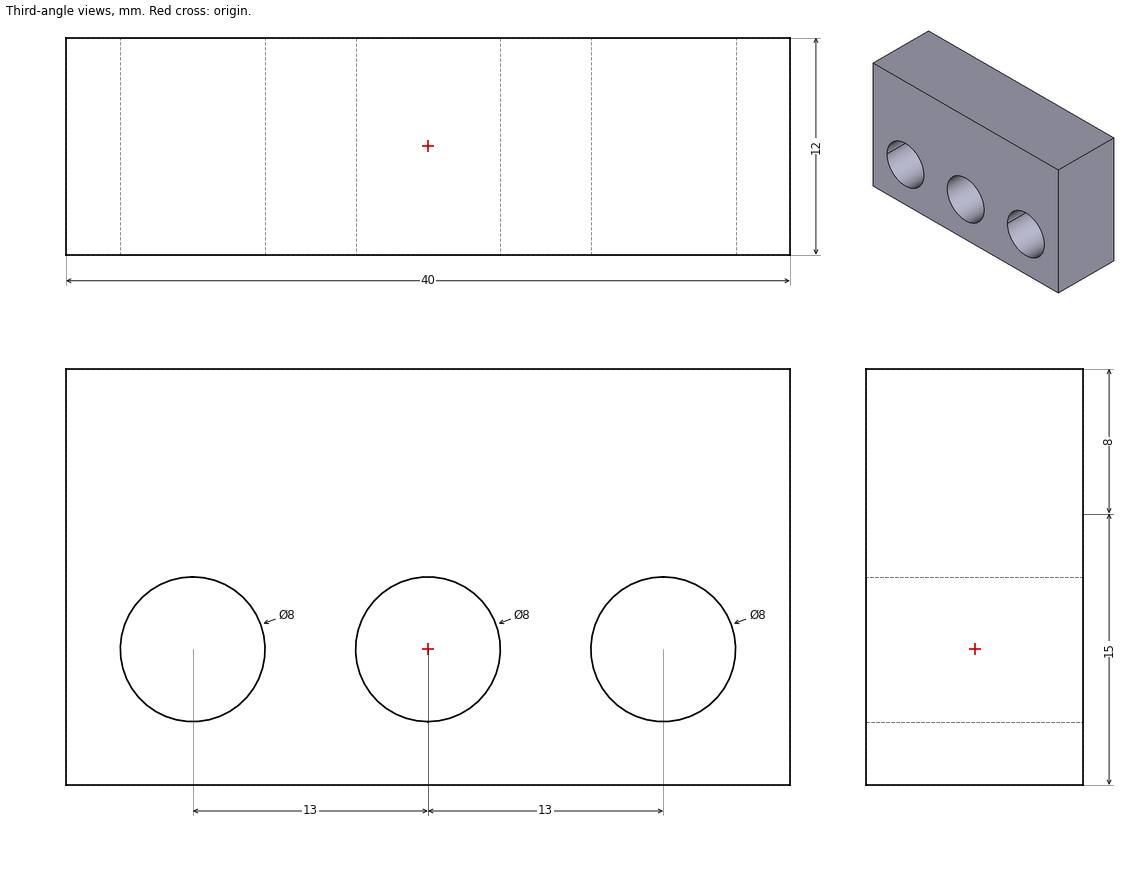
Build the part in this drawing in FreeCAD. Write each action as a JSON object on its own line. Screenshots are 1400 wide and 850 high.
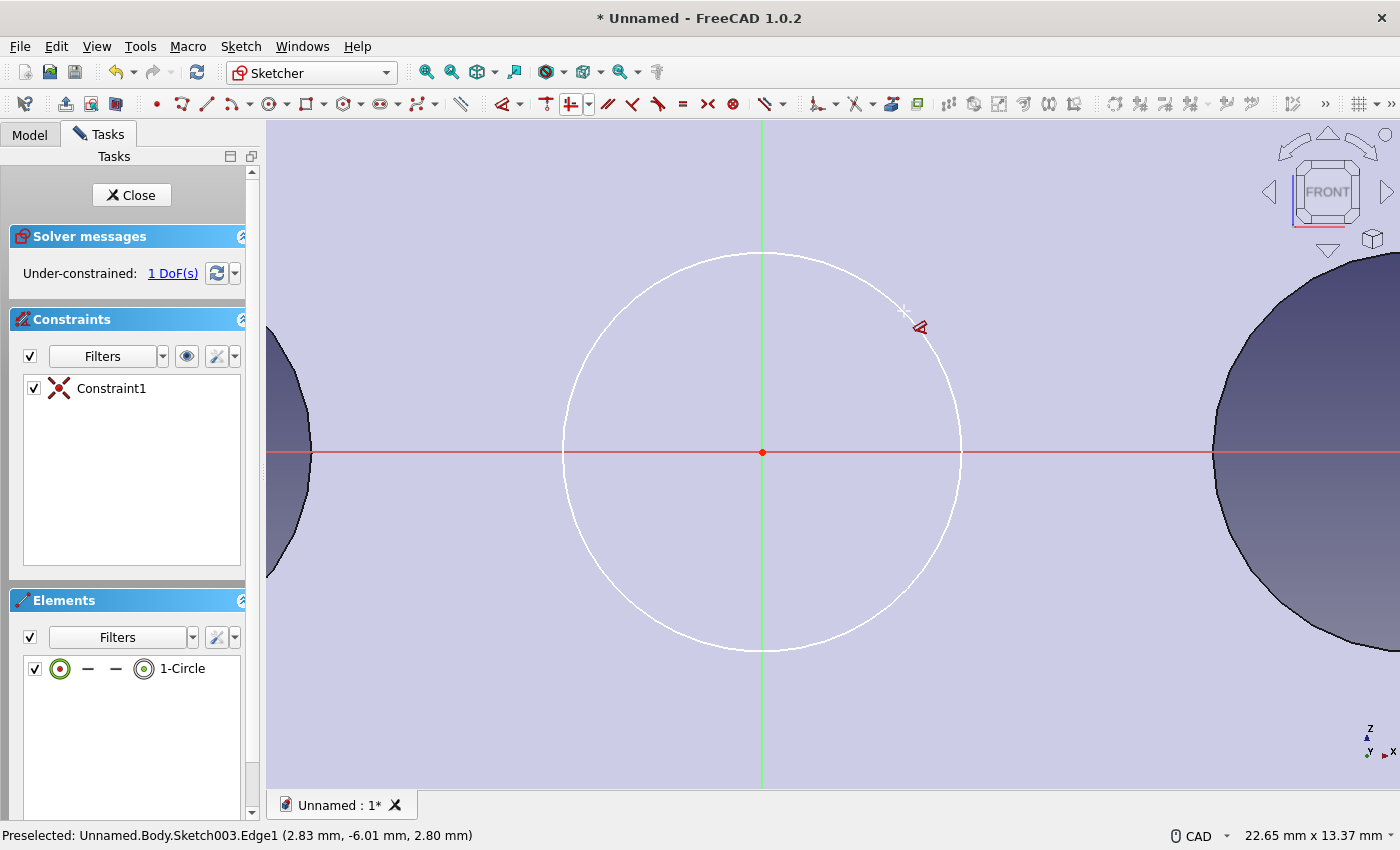
{"action": "left_click", "coordinate": [903, 311]}
{"action": "left_click", "coordinate": [926, 288]}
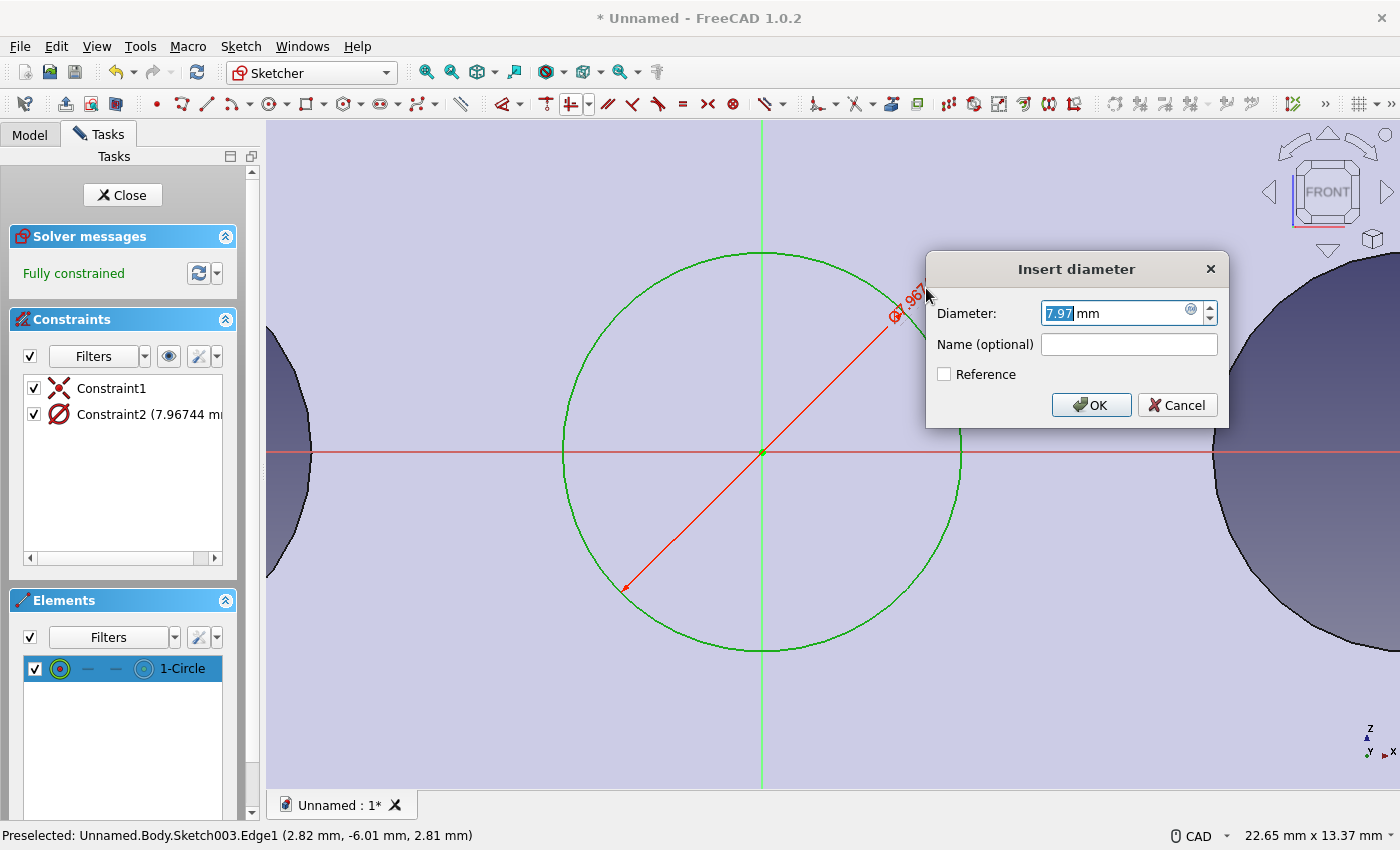
{"action": "type", "text": "8"}
{"action": "key", "text": "Return"}
{"action": "key", "text": "Escape"}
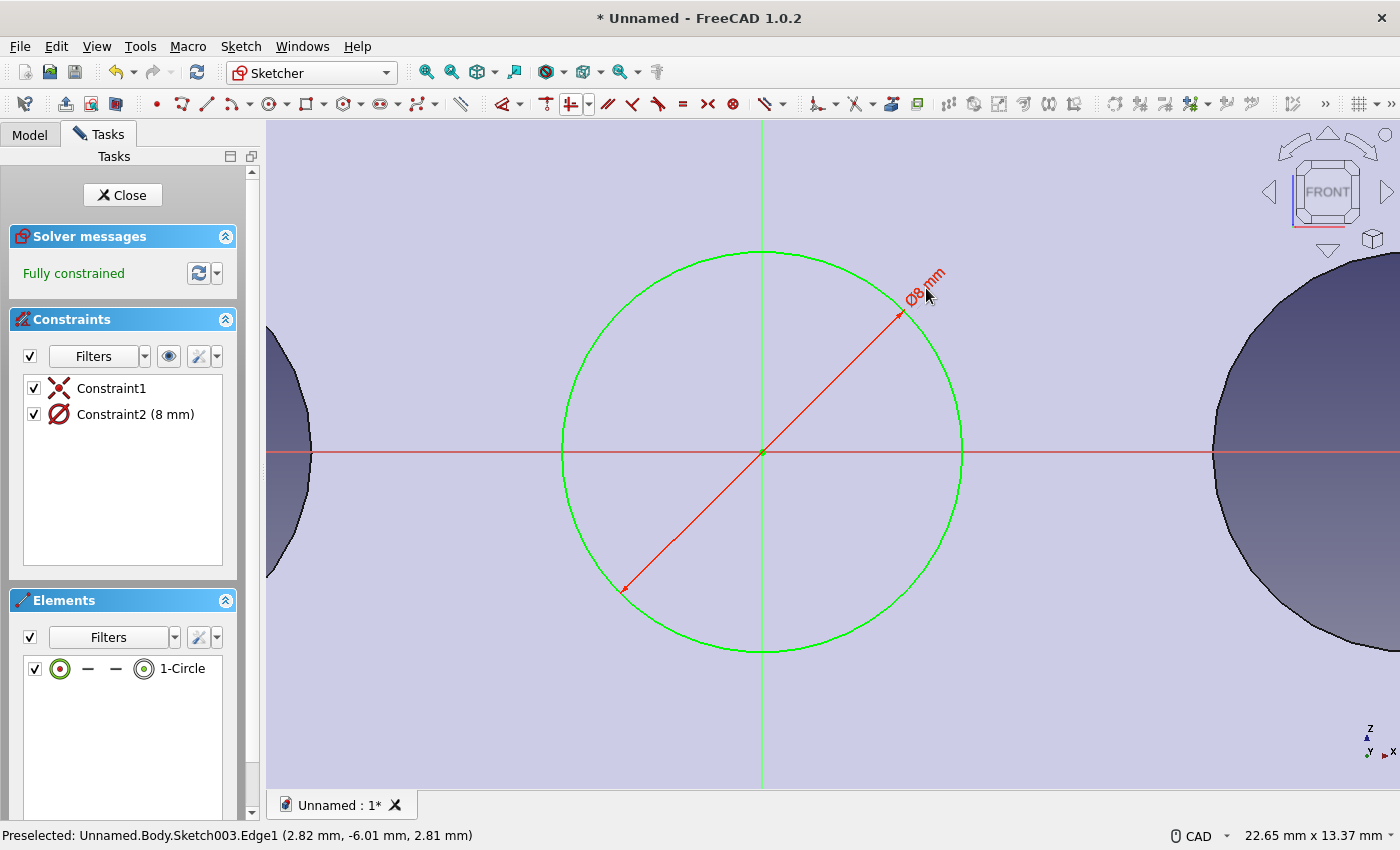
{"action": "left_click", "coordinate": [123, 195]}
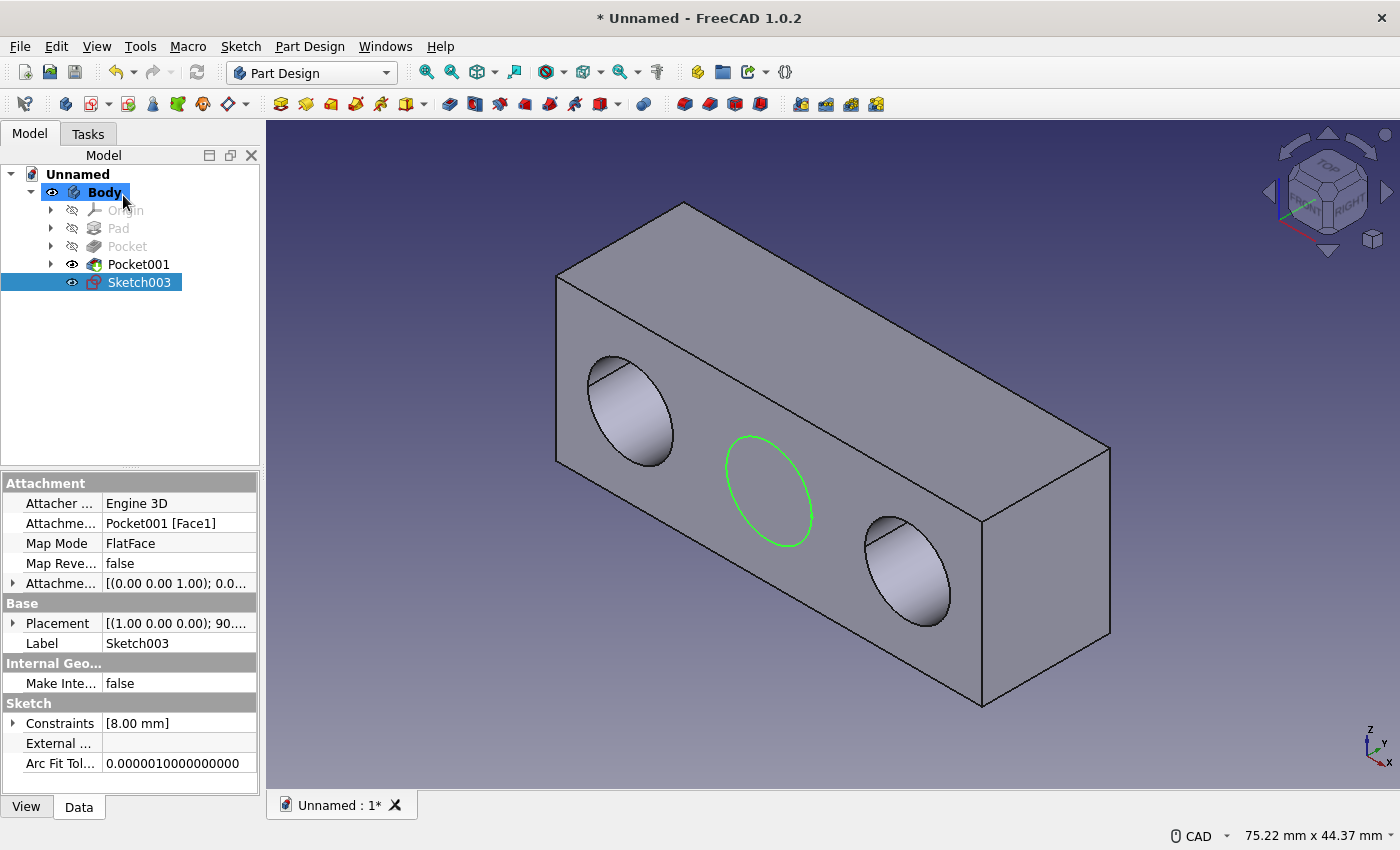
{"action": "left_click", "coordinate": [450, 104]}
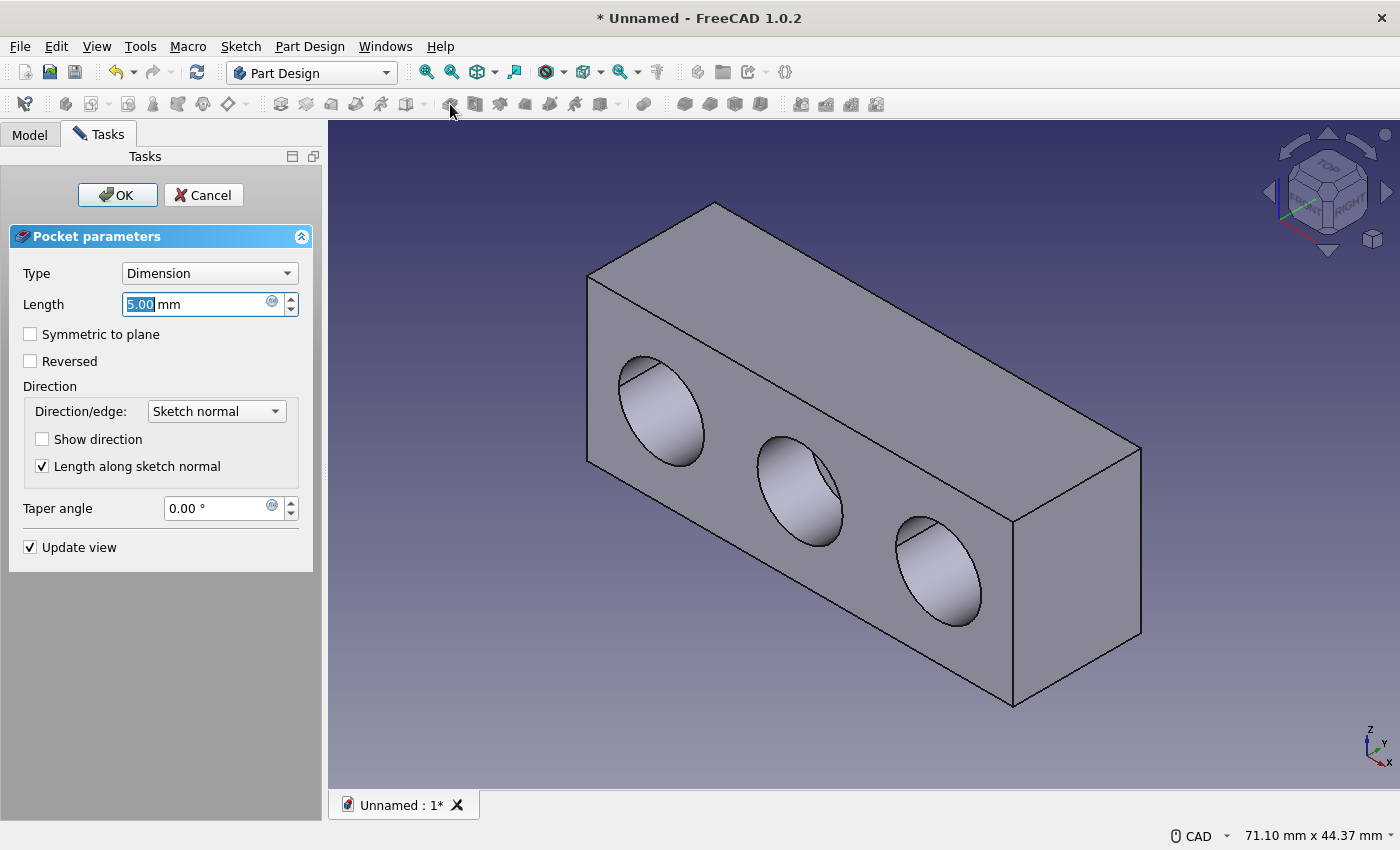
{"action": "left_click", "coordinate": [210, 274]}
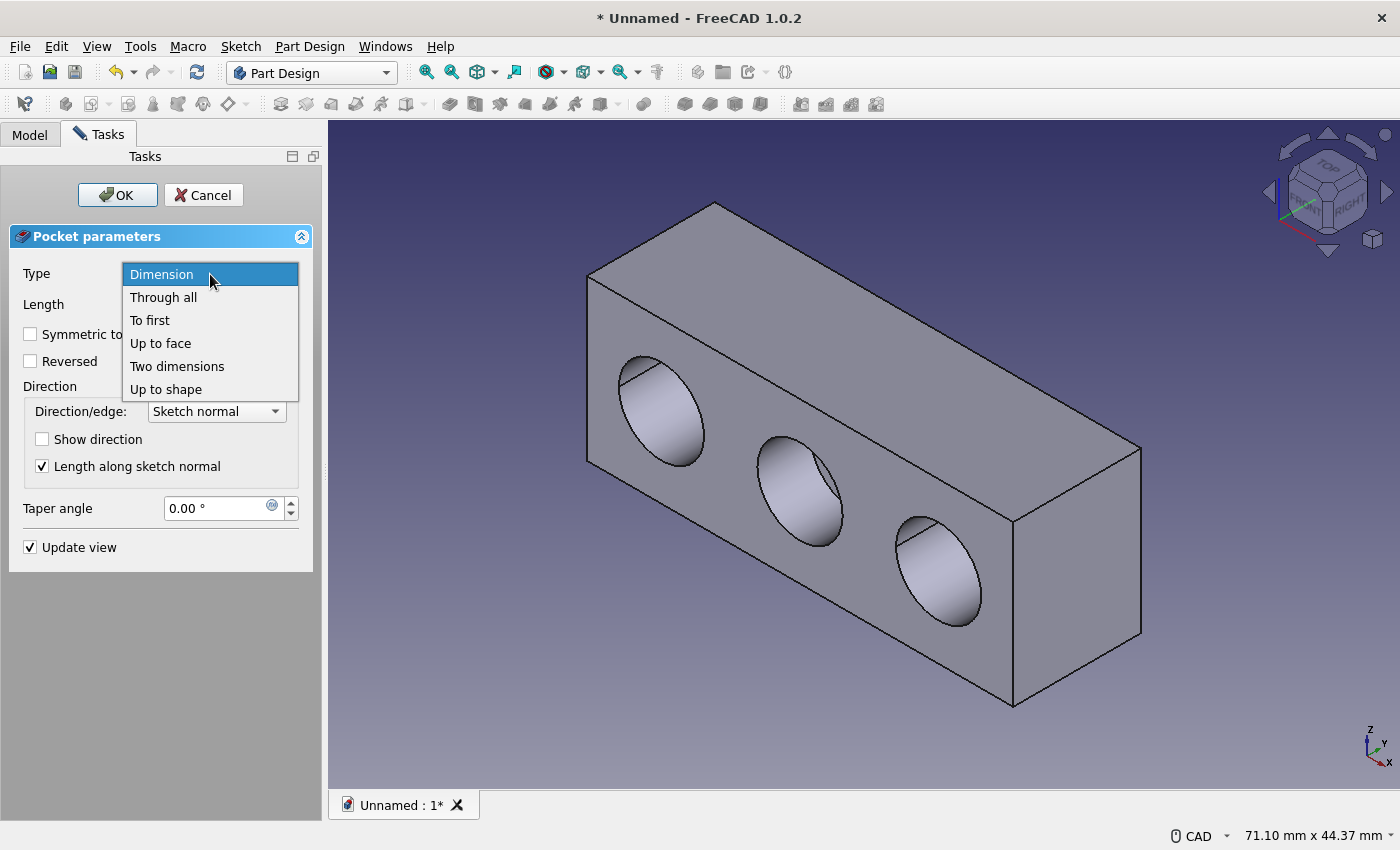
{"action": "left_click", "coordinate": [208, 320]}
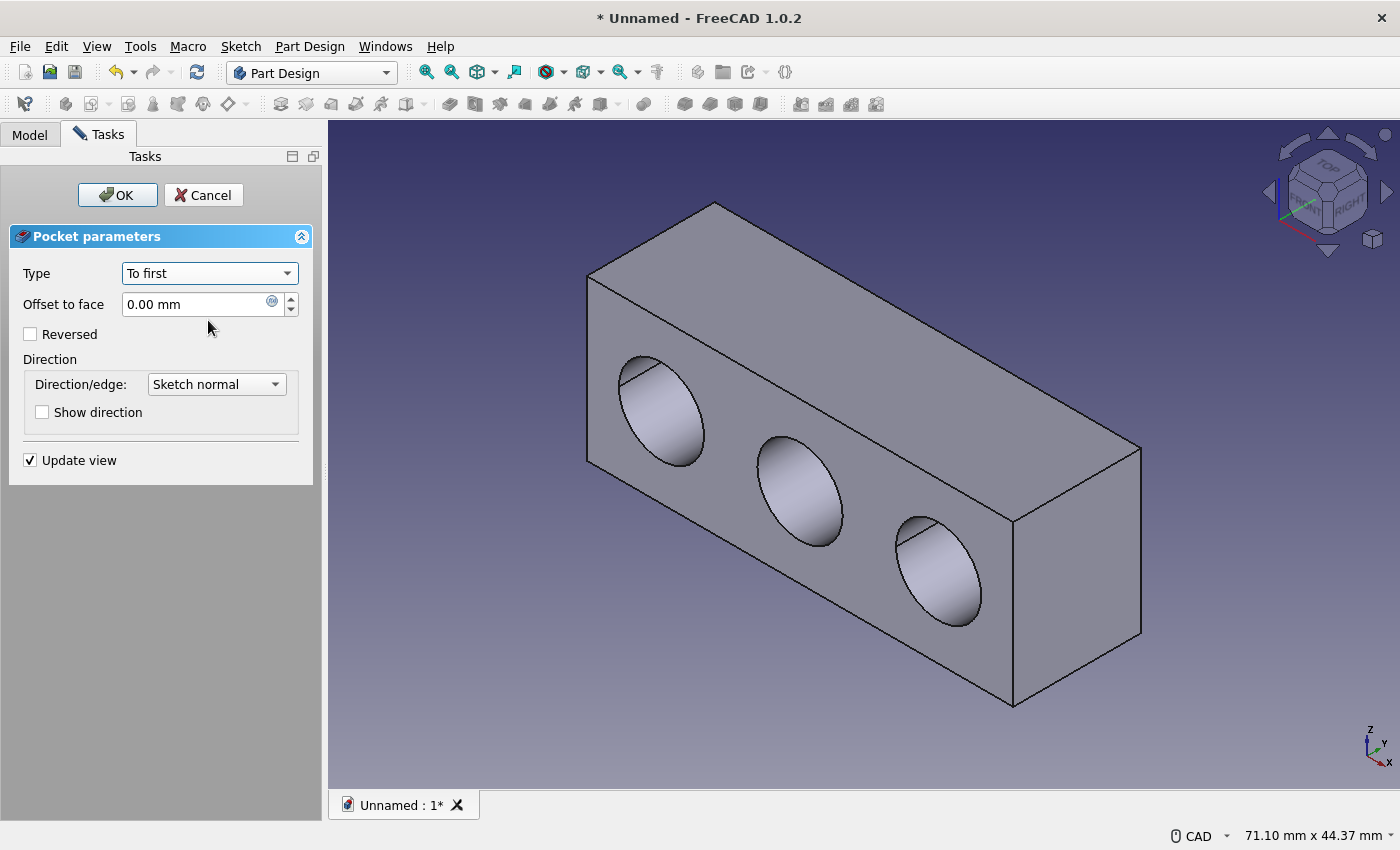
{"action": "left_click", "coordinate": [118, 195]}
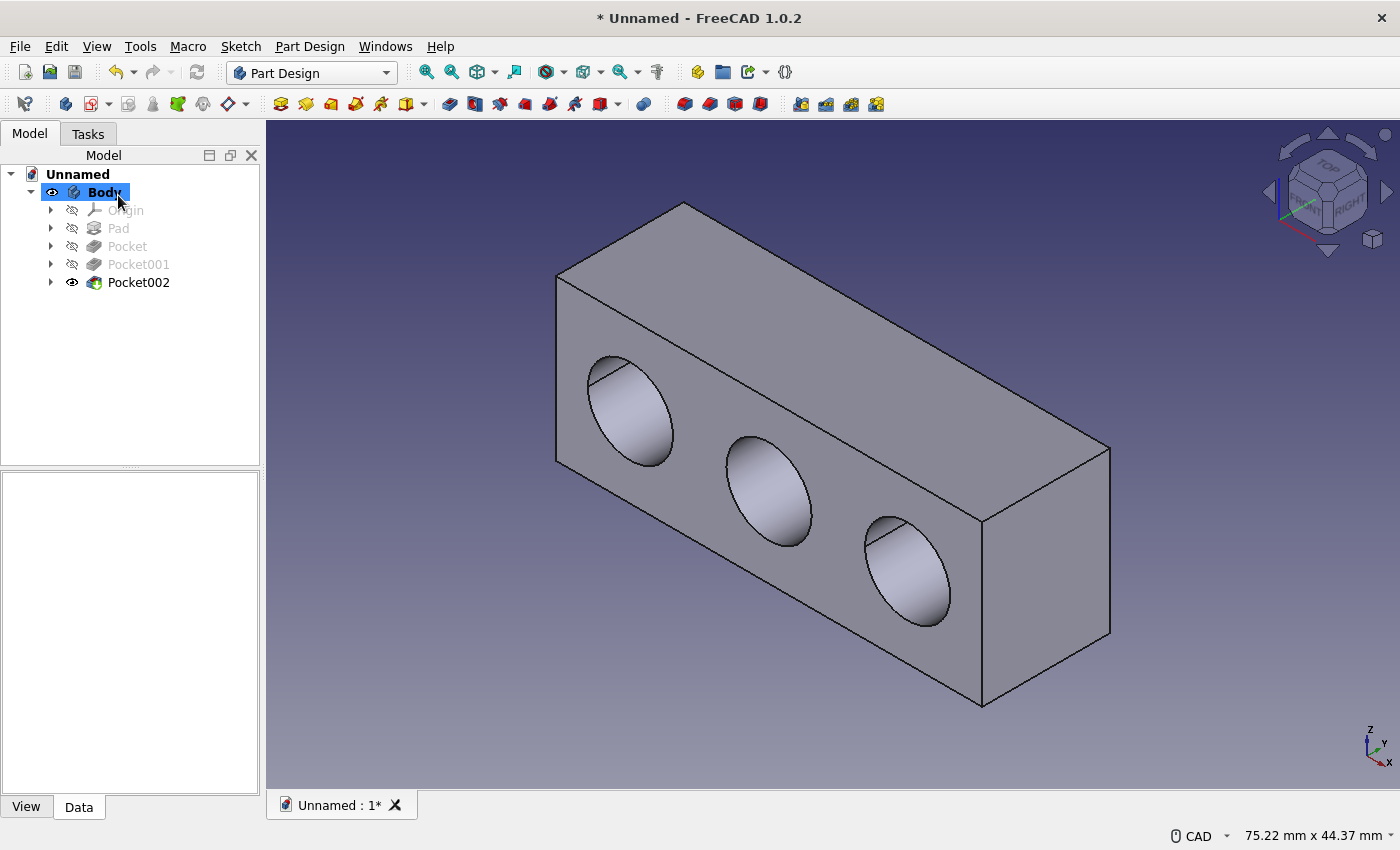
{"action": "left_click", "coordinate": [955, 432]}